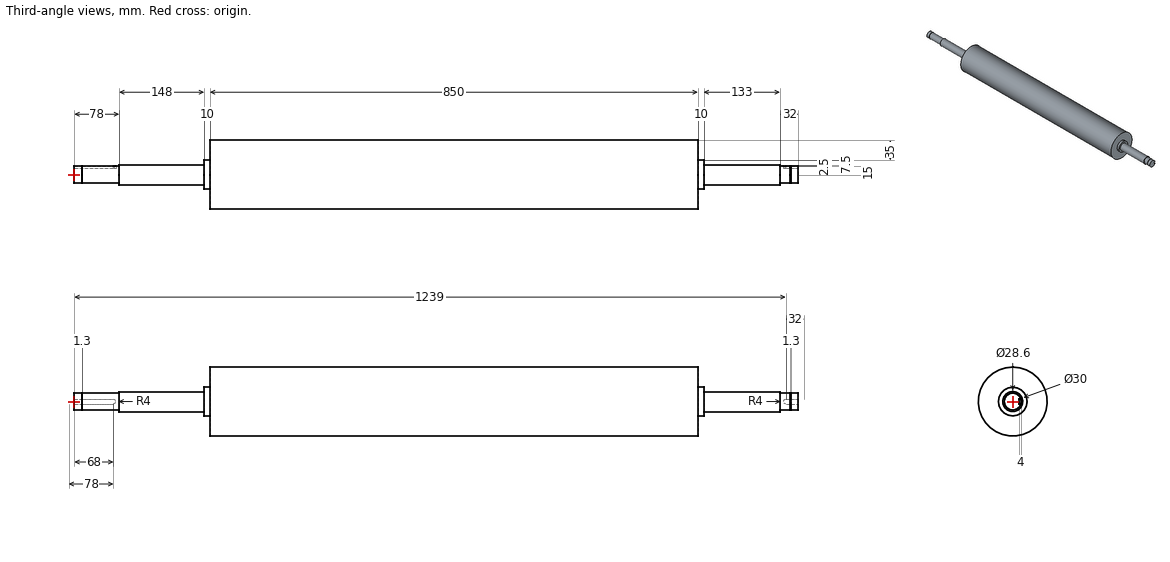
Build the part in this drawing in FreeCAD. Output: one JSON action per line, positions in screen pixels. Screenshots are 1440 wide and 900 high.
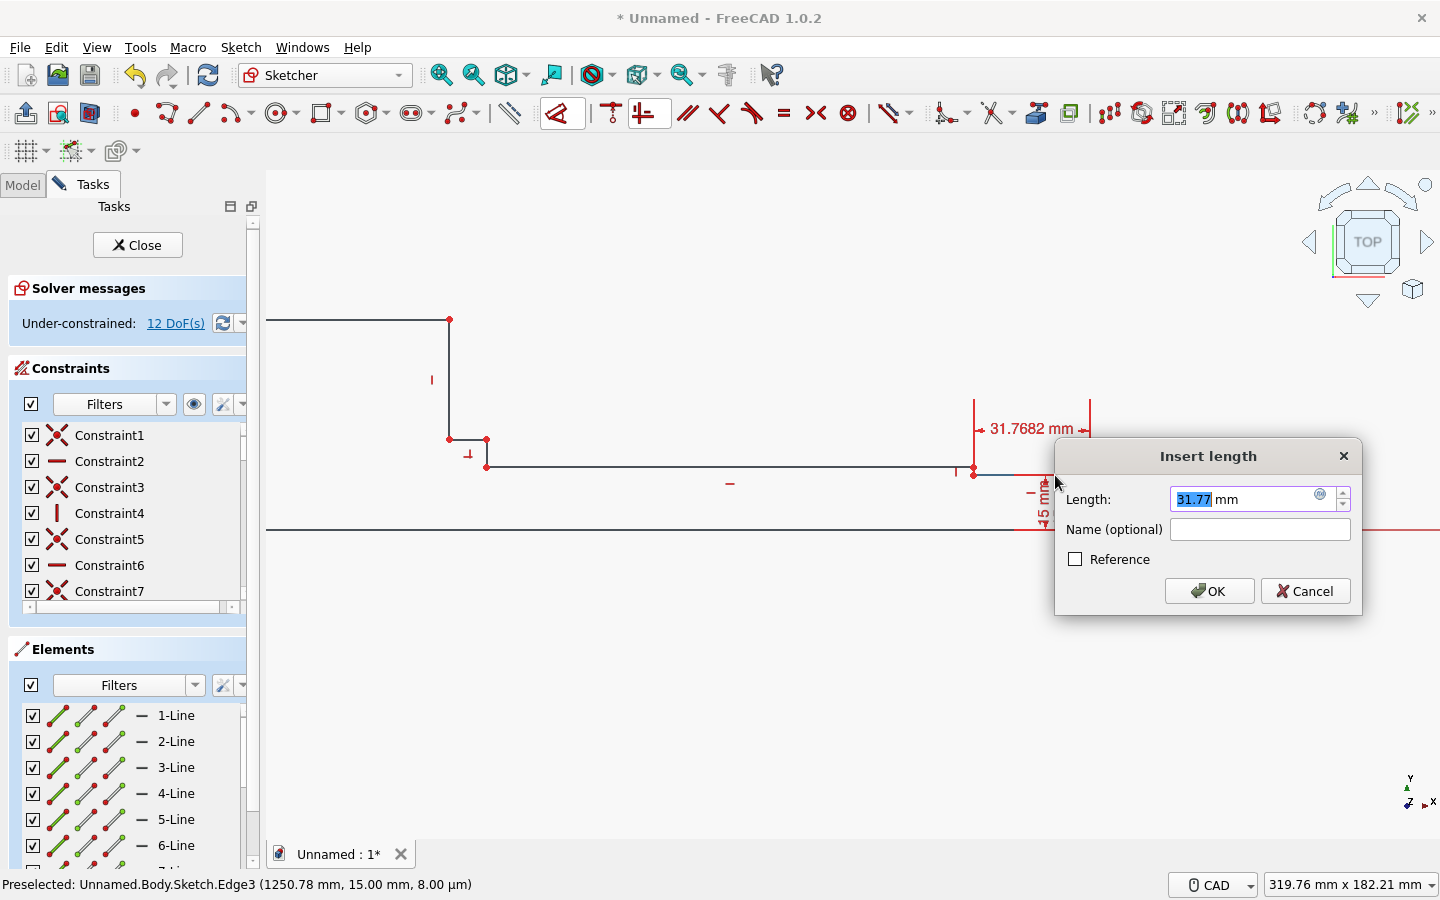
{"action": "type", "text": "32"}
{"action": "key", "text": "Return"}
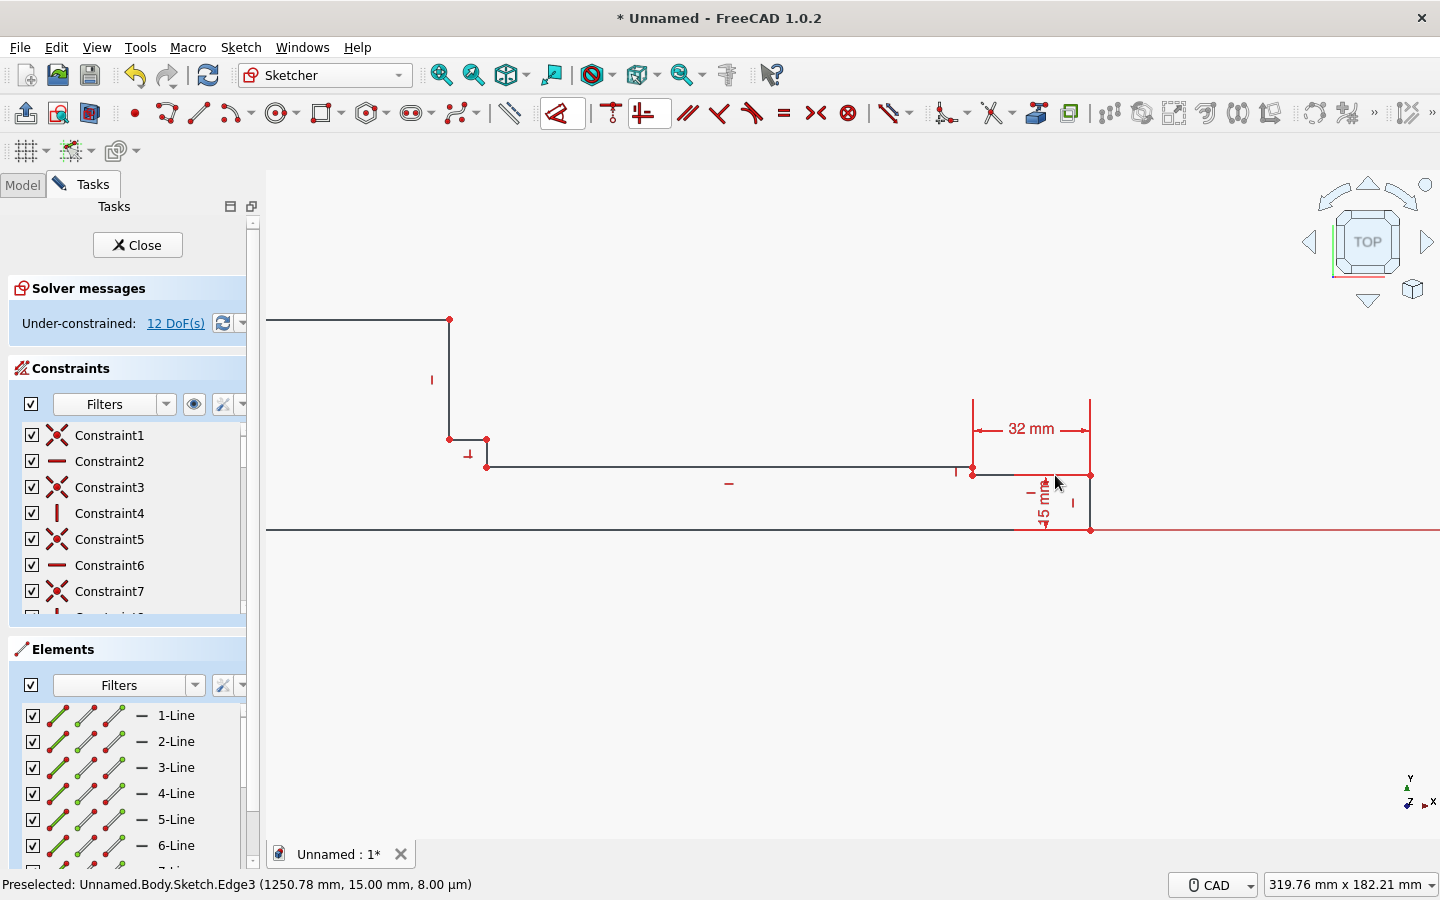
{"action": "scroll", "coordinate": [476, 440], "scroll_direction": "up", "scroll_amount": 2}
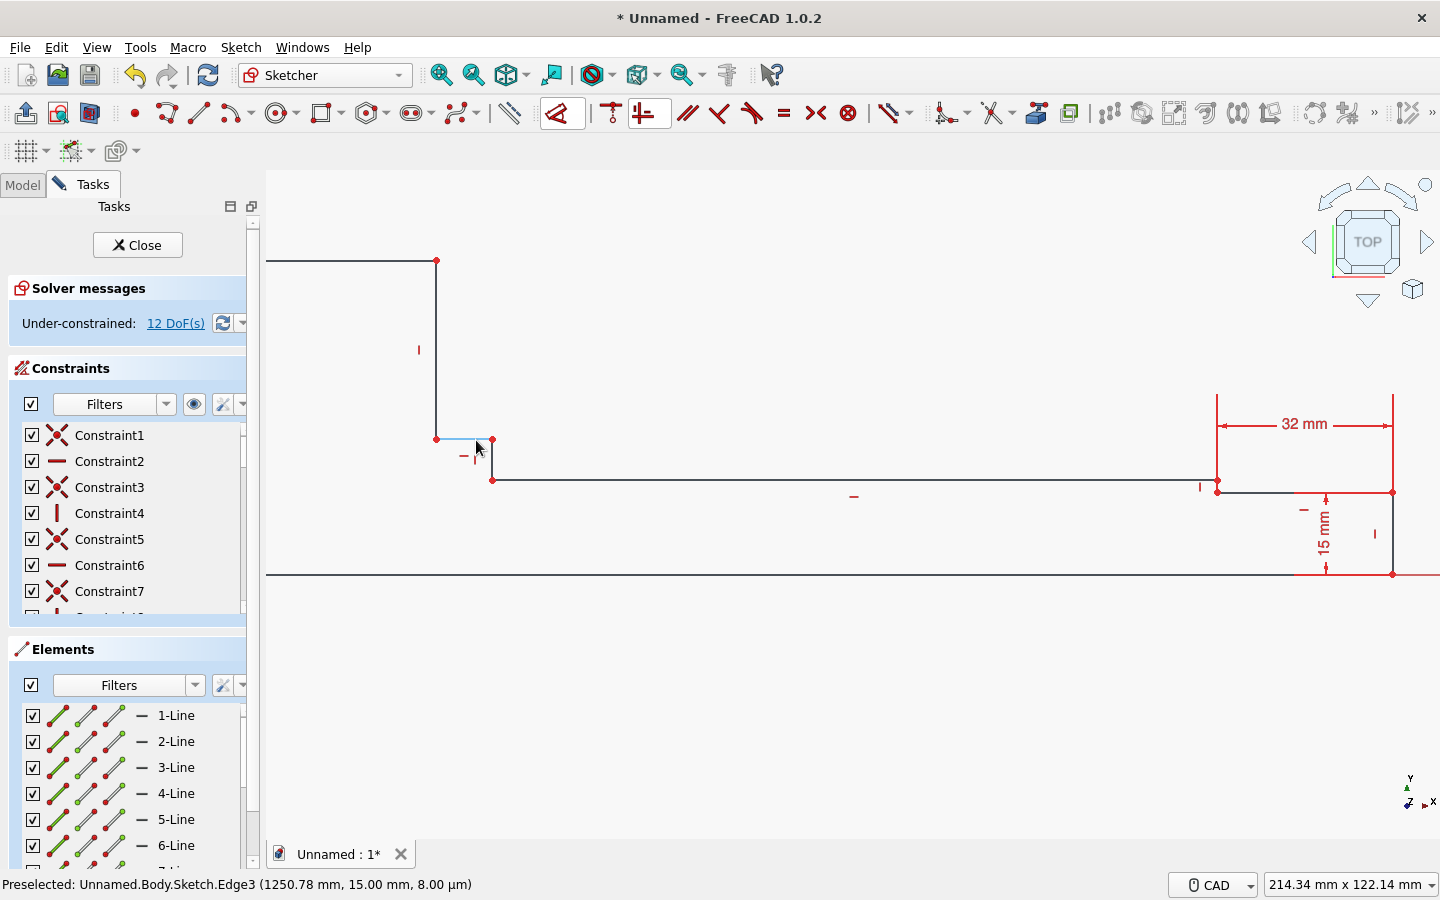
{"action": "left_click", "coordinate": [475, 439]}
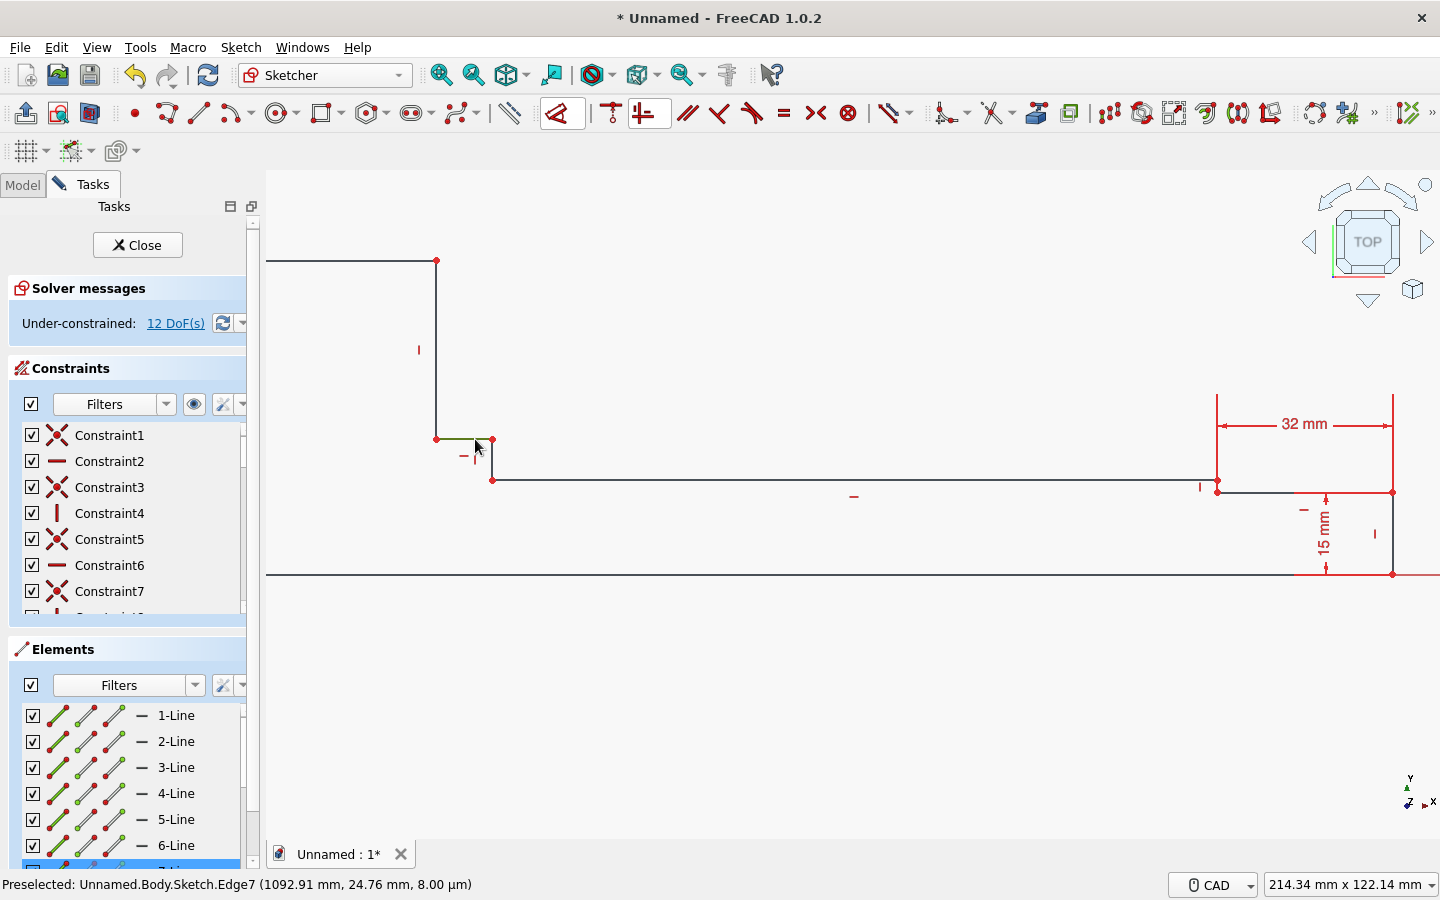
{"action": "left_click", "coordinate": [580, 114]}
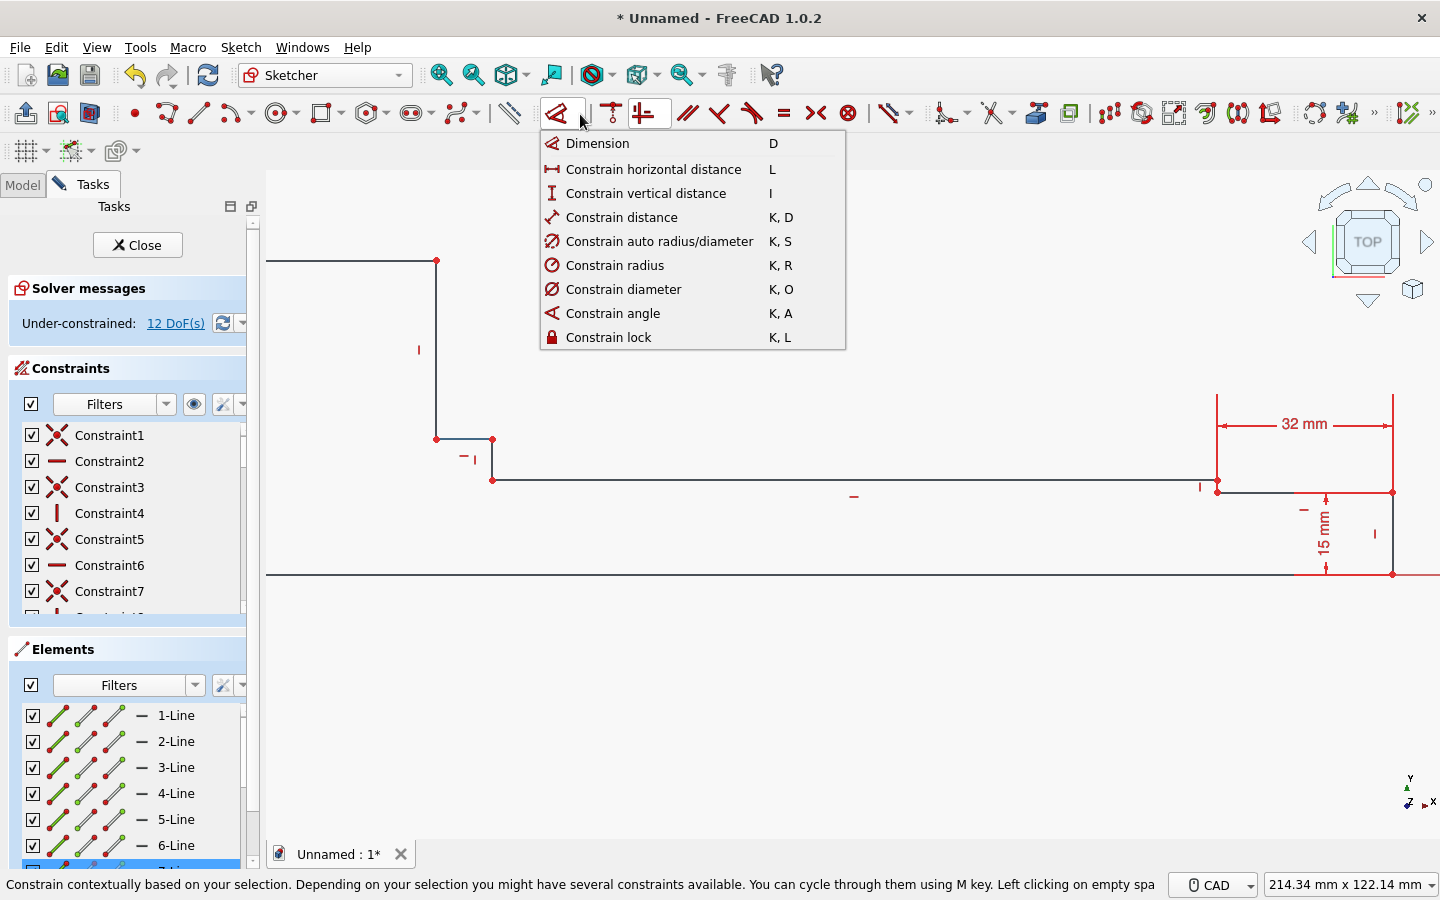
{"action": "left_click", "coordinate": [693, 169]}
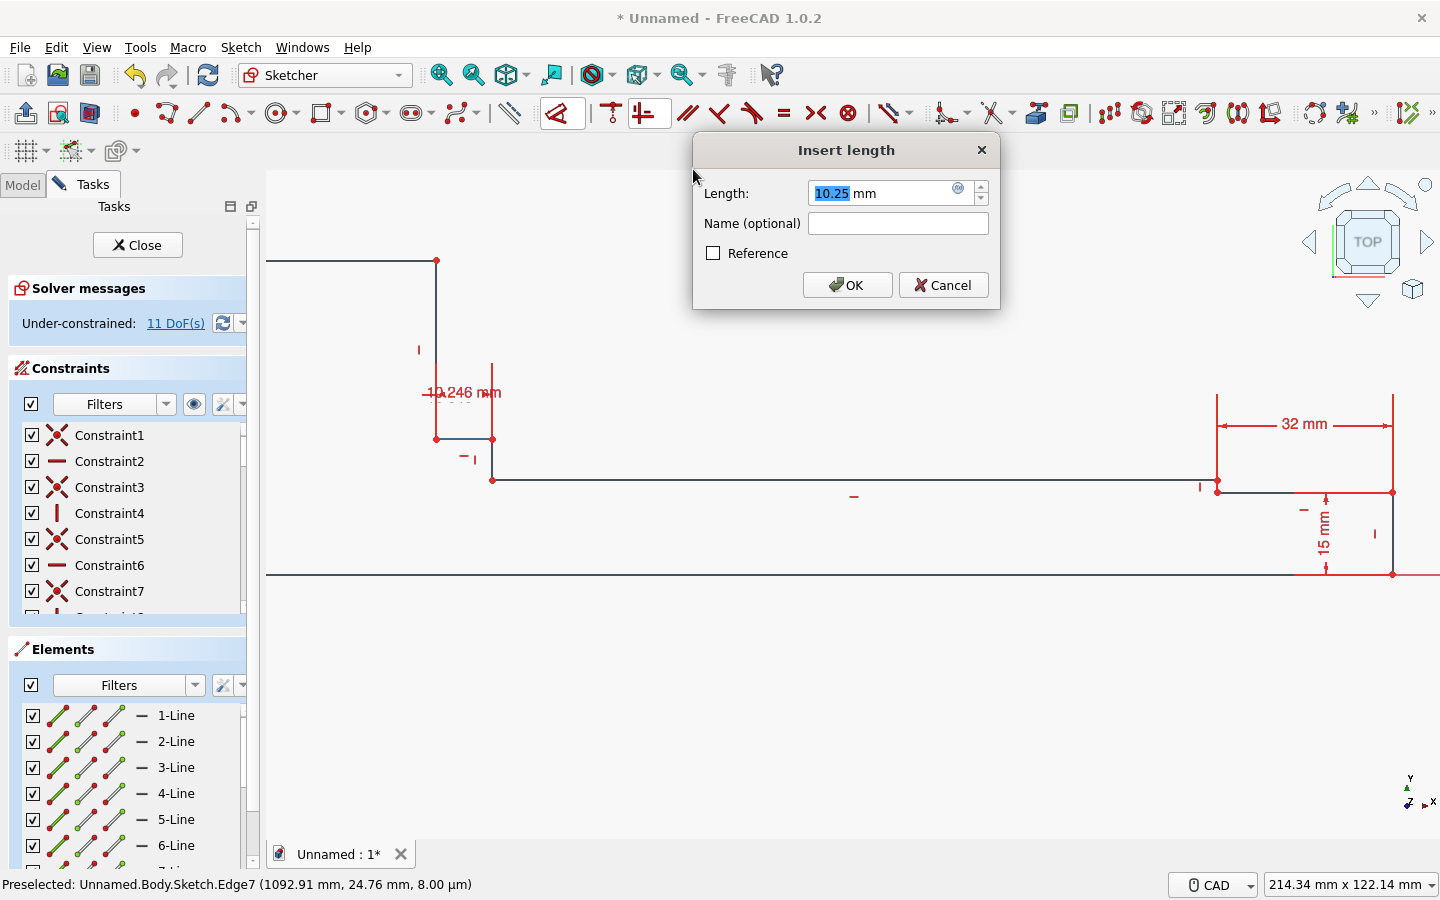
{"action": "type", "text": "10"}
{"action": "key", "text": "Return"}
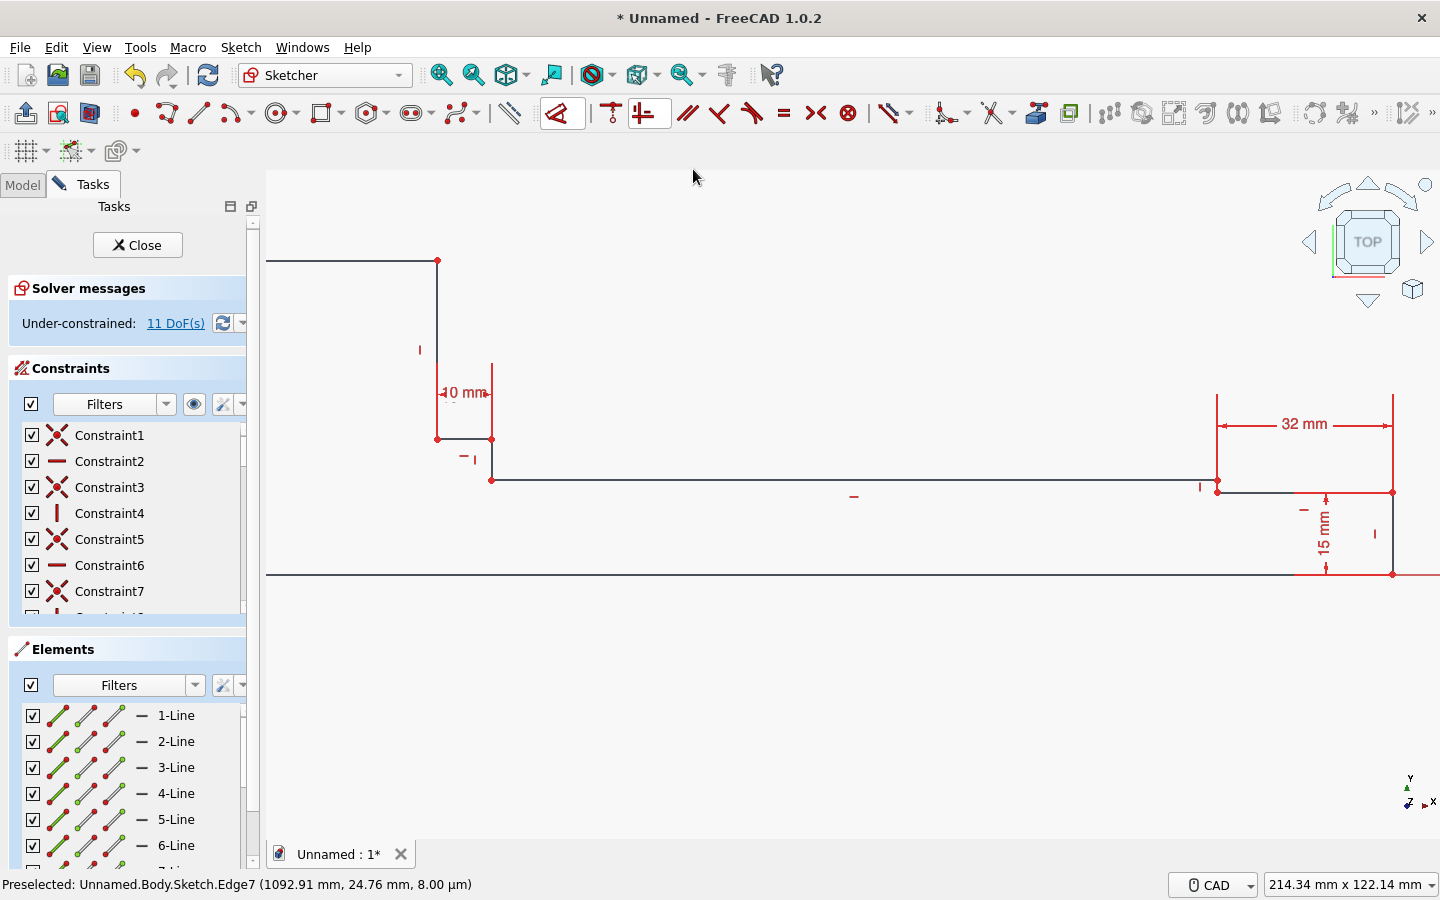
{"action": "scroll", "coordinate": [1068, 514], "scroll_direction": "down", "scroll_amount": 12}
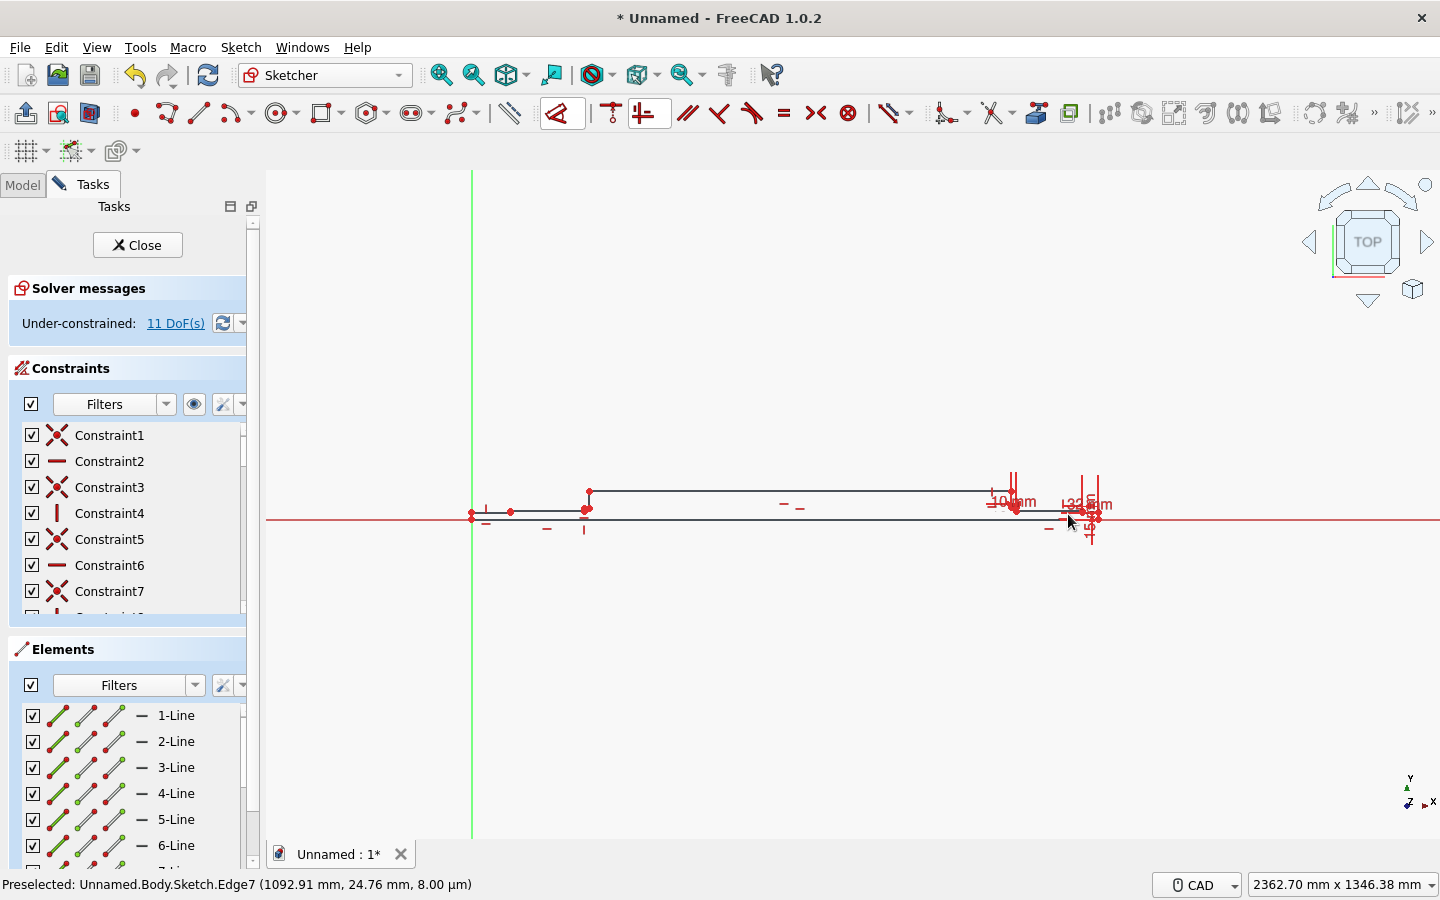
{"action": "scroll", "coordinate": [1011, 503], "scroll_direction": "up", "scroll_amount": 6}